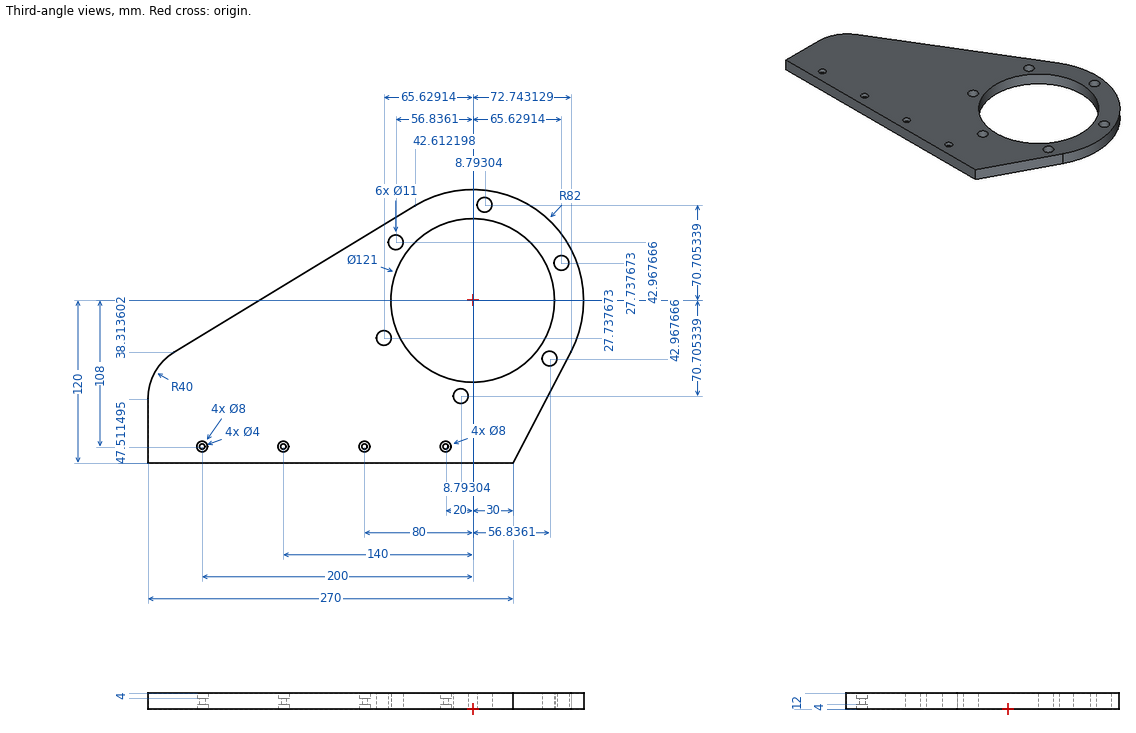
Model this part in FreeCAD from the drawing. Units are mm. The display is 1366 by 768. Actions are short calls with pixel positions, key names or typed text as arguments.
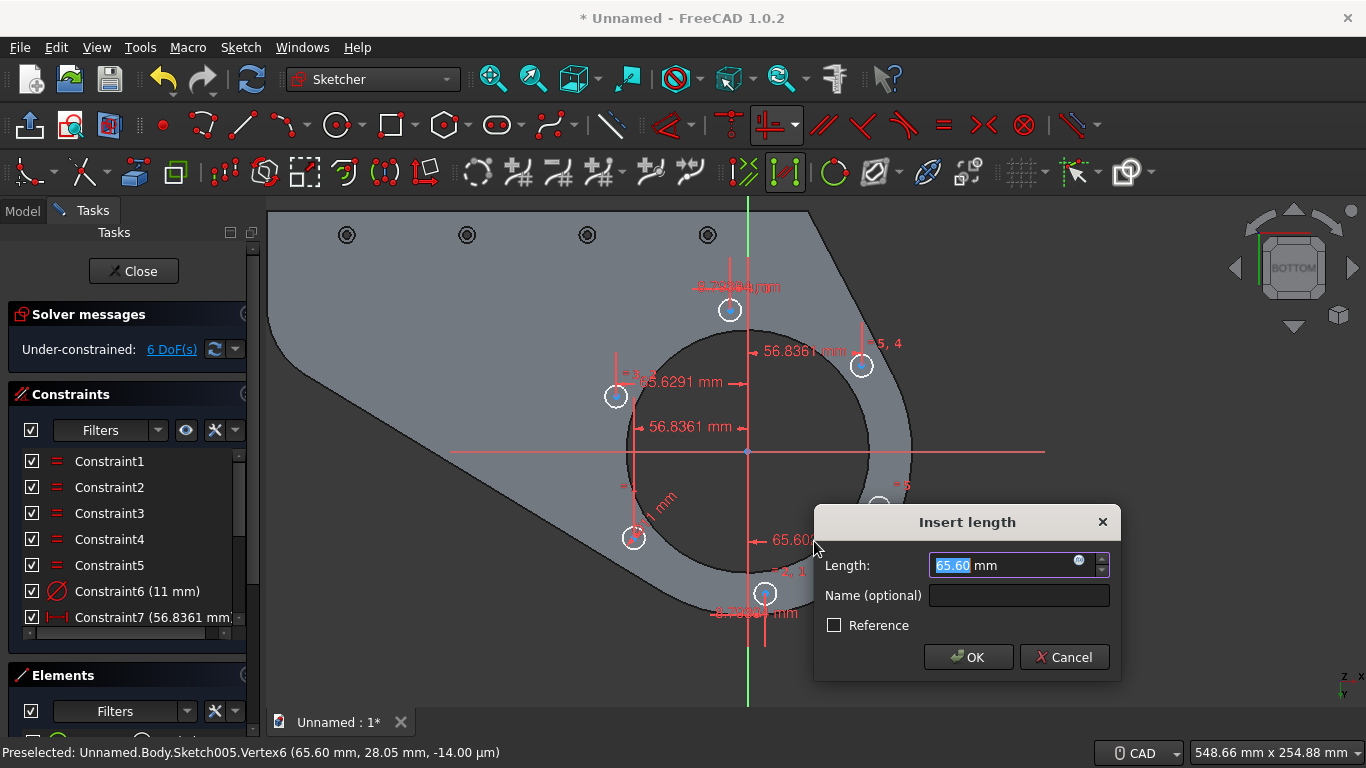
text(65.62914)
key(Return)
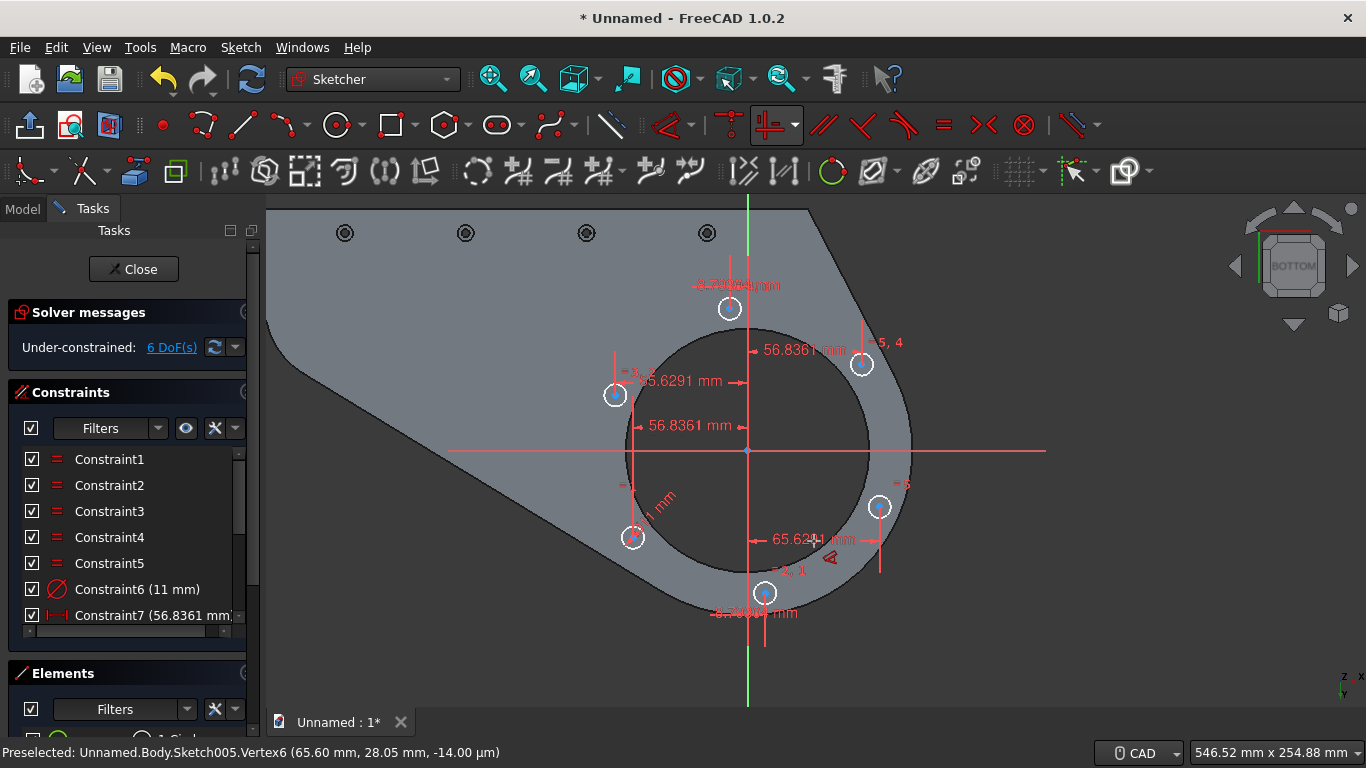
click(633, 538)
click(599, 474)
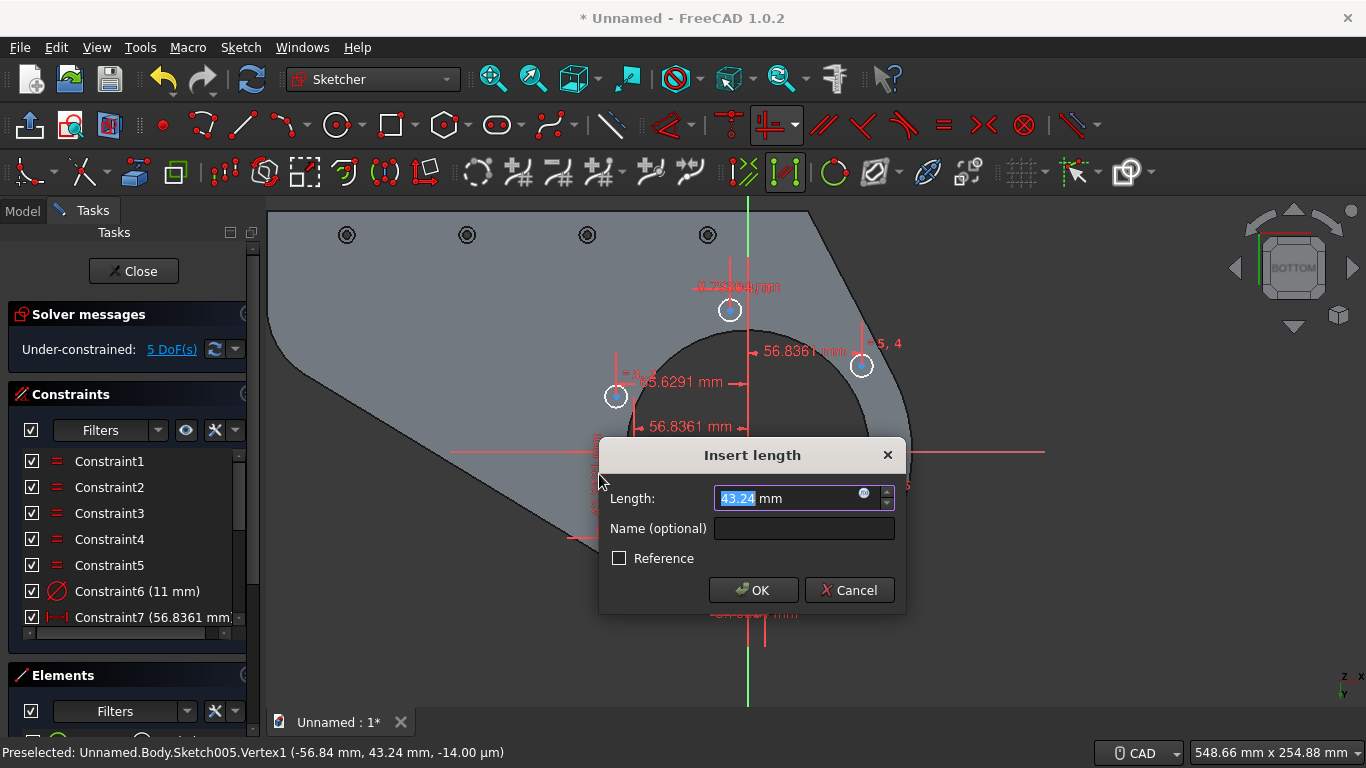
text(42.967666)
key(Return)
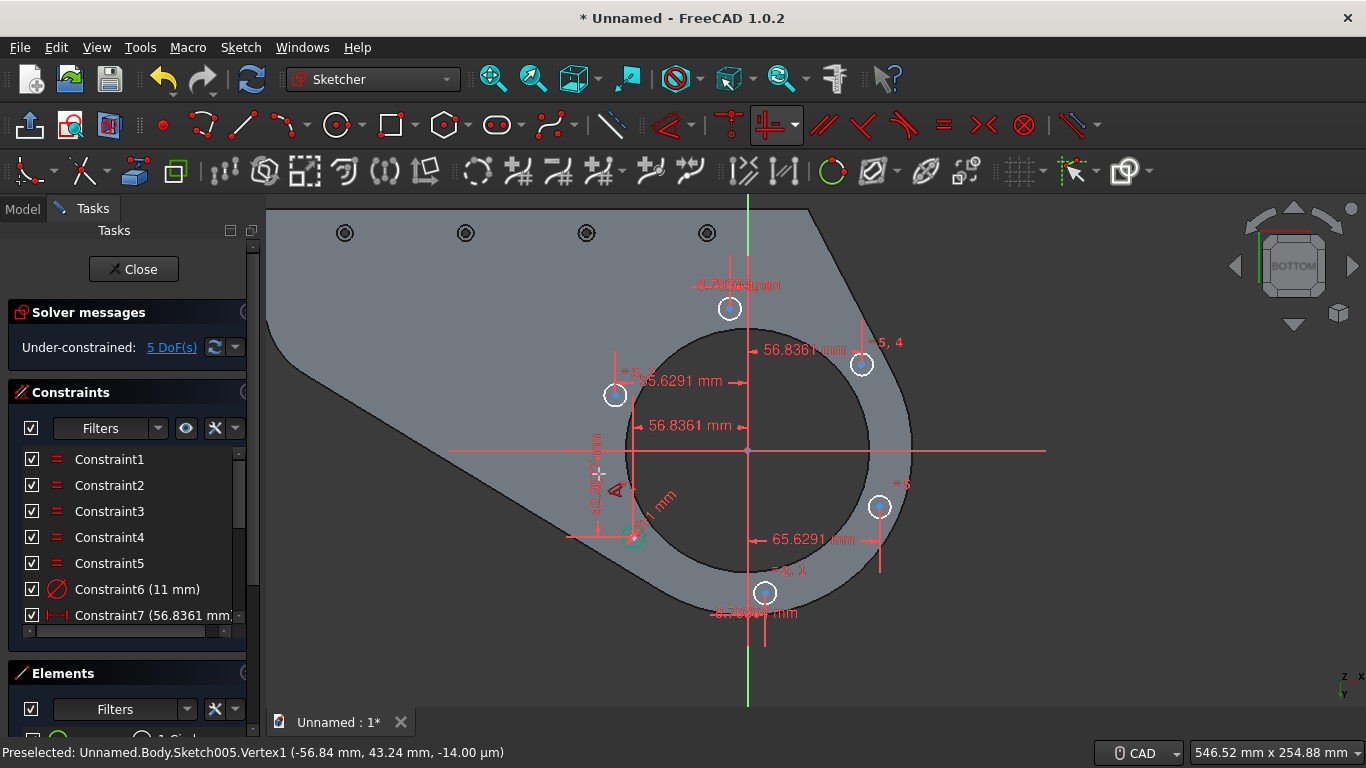
click(765, 593)
click(799, 489)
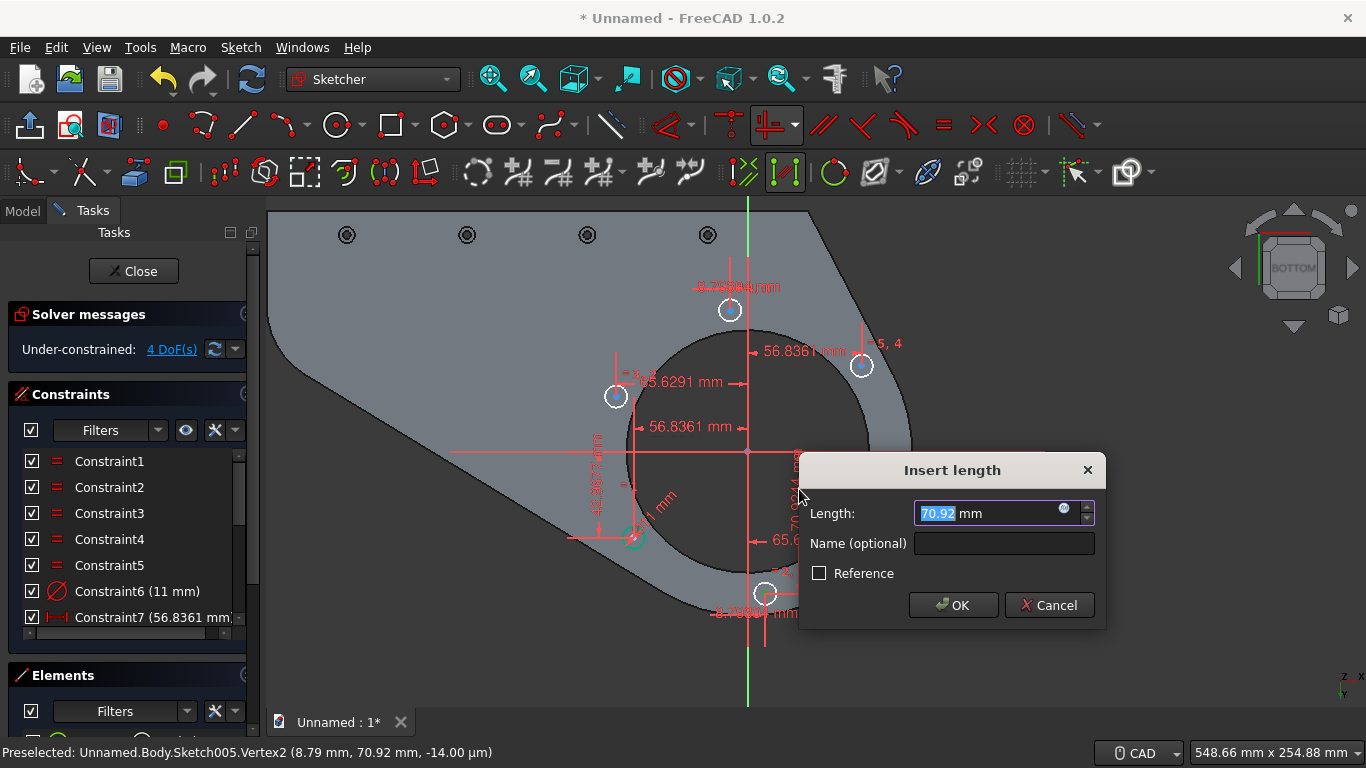
text(70.705339)
key(Return)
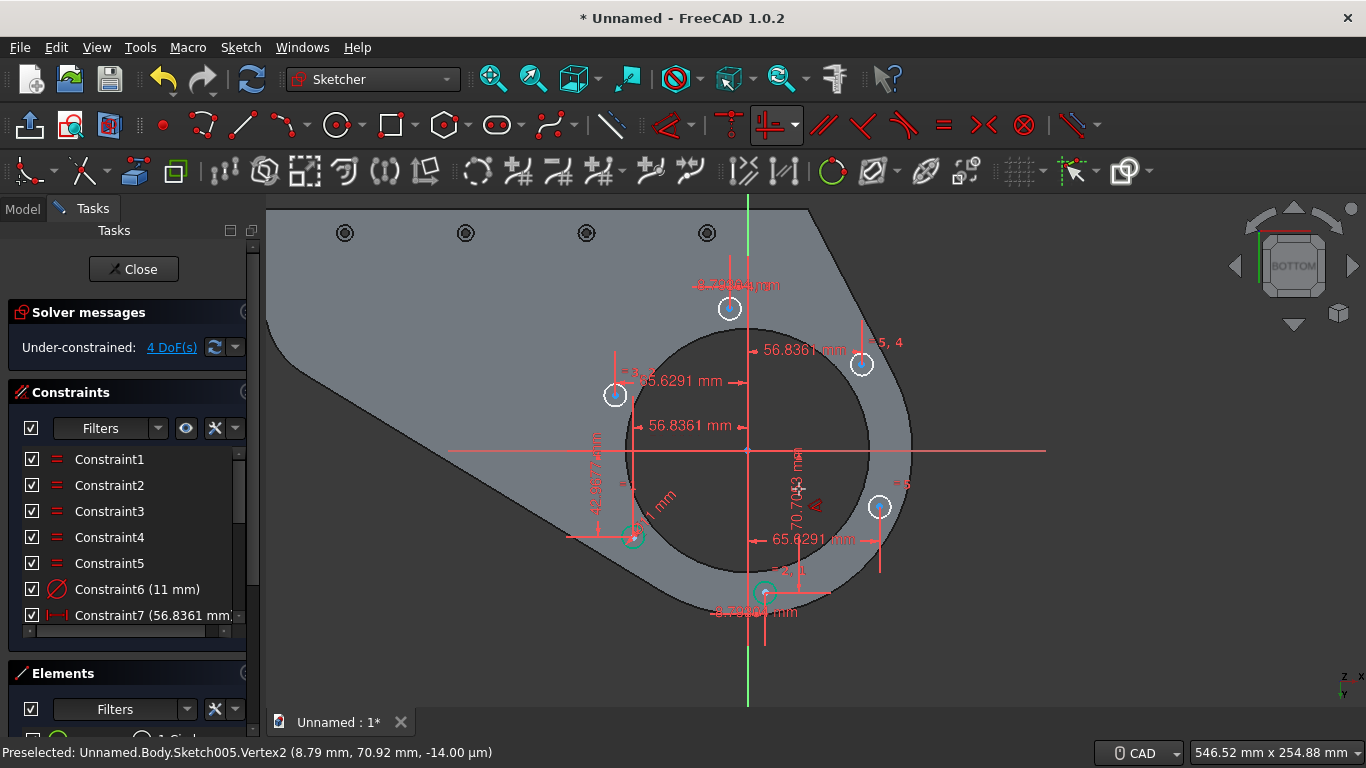
click(615, 395)
click(581, 423)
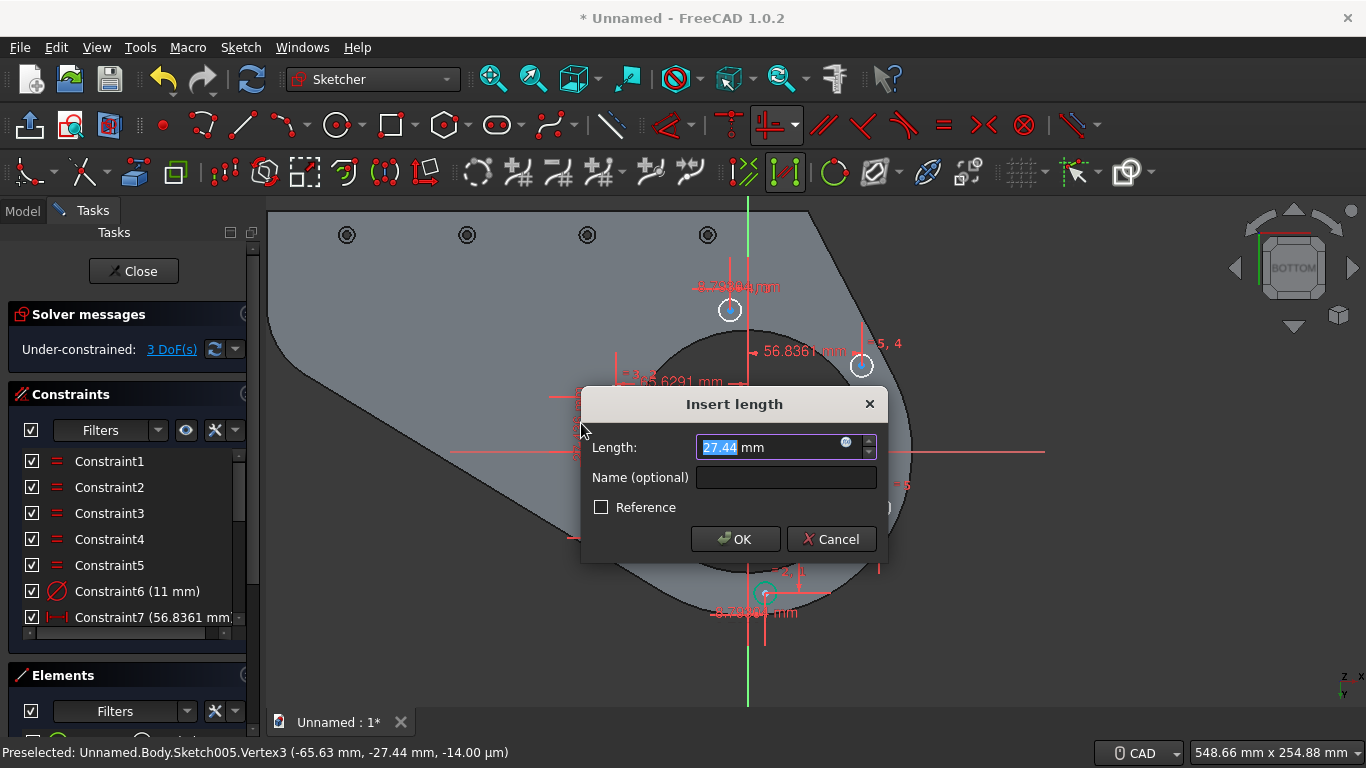
text(27.737673)
key(Return)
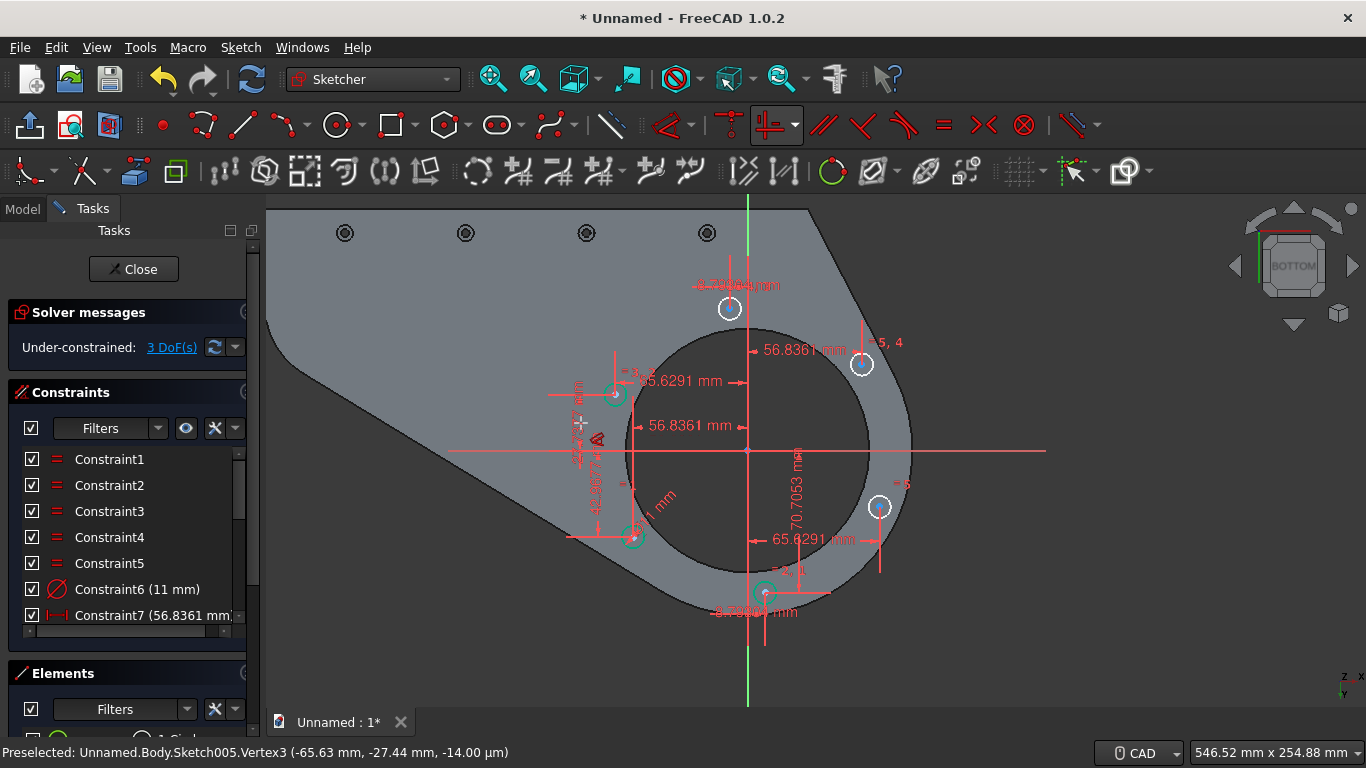
click(730, 309)
click(696, 347)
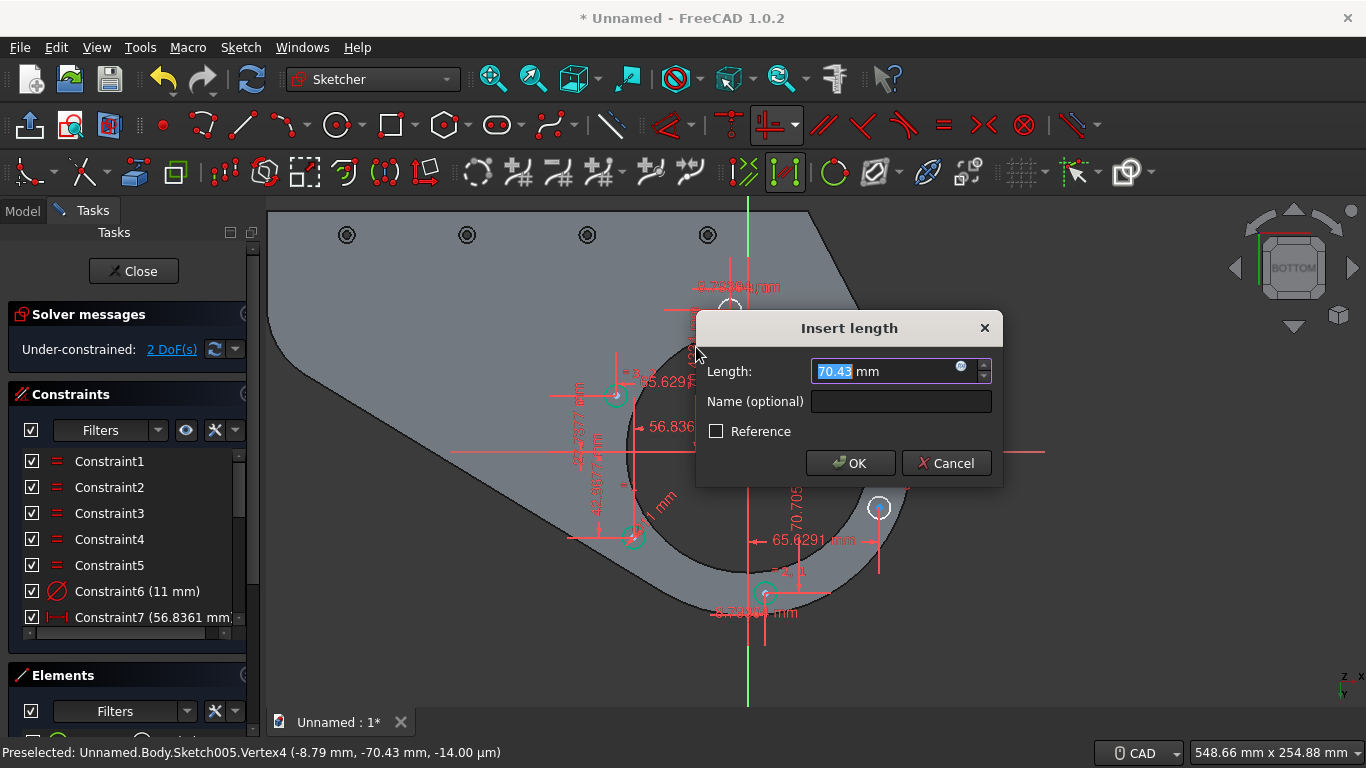
text(70.705339)
key(Return)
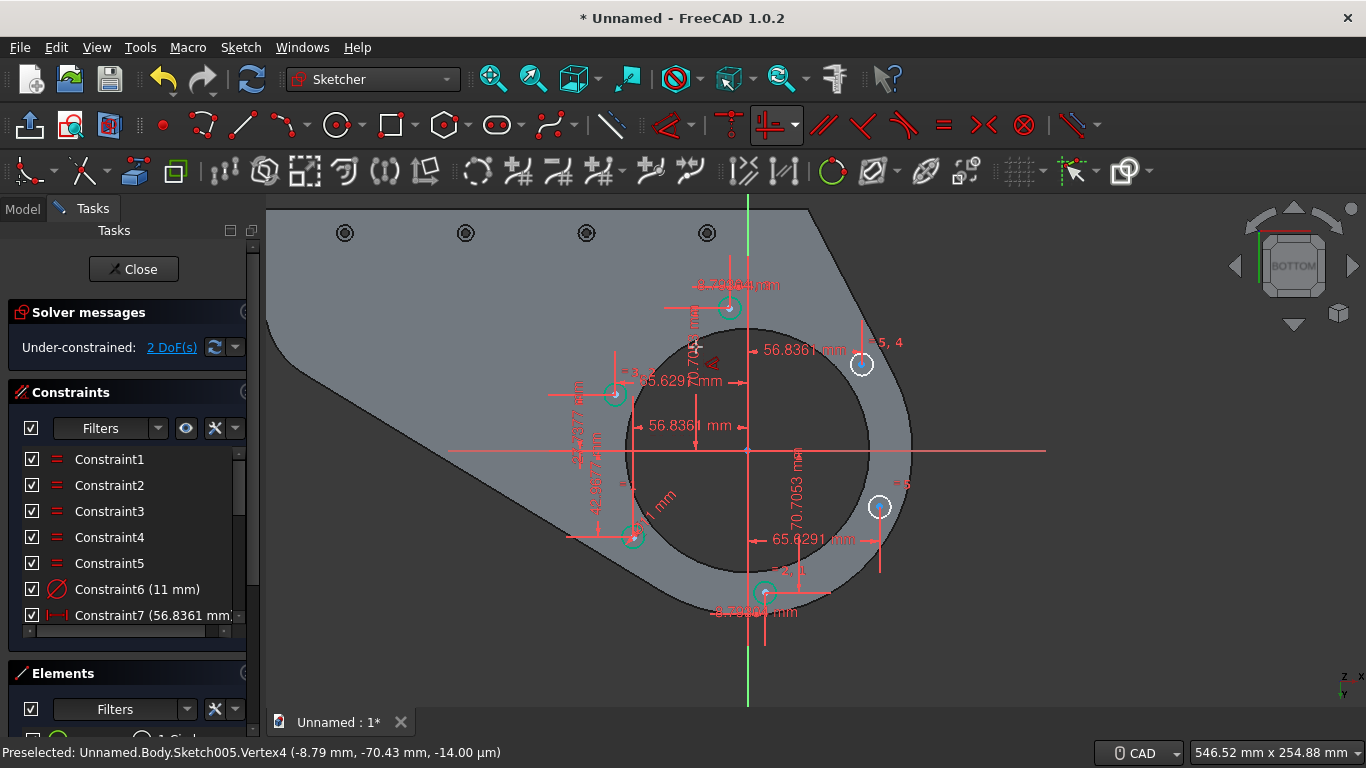
click(862, 364)
click(896, 408)